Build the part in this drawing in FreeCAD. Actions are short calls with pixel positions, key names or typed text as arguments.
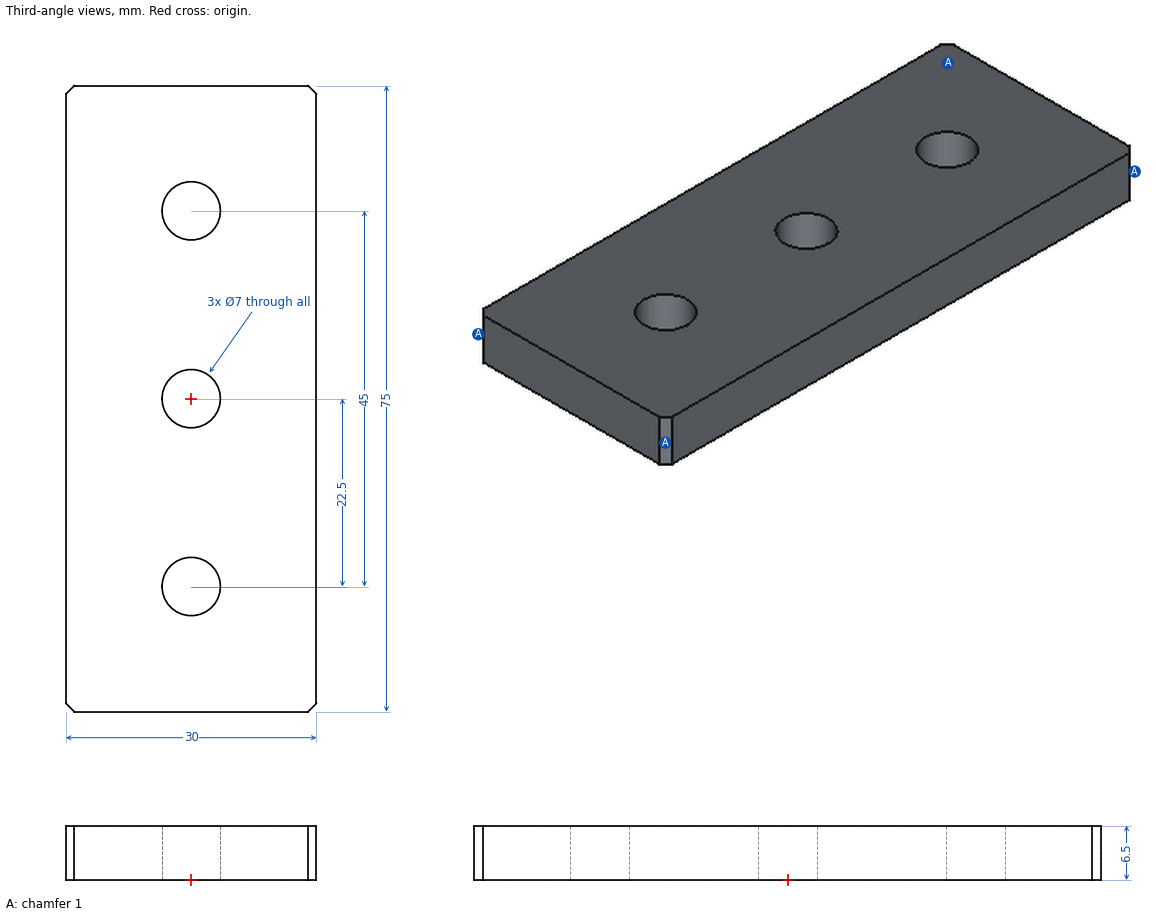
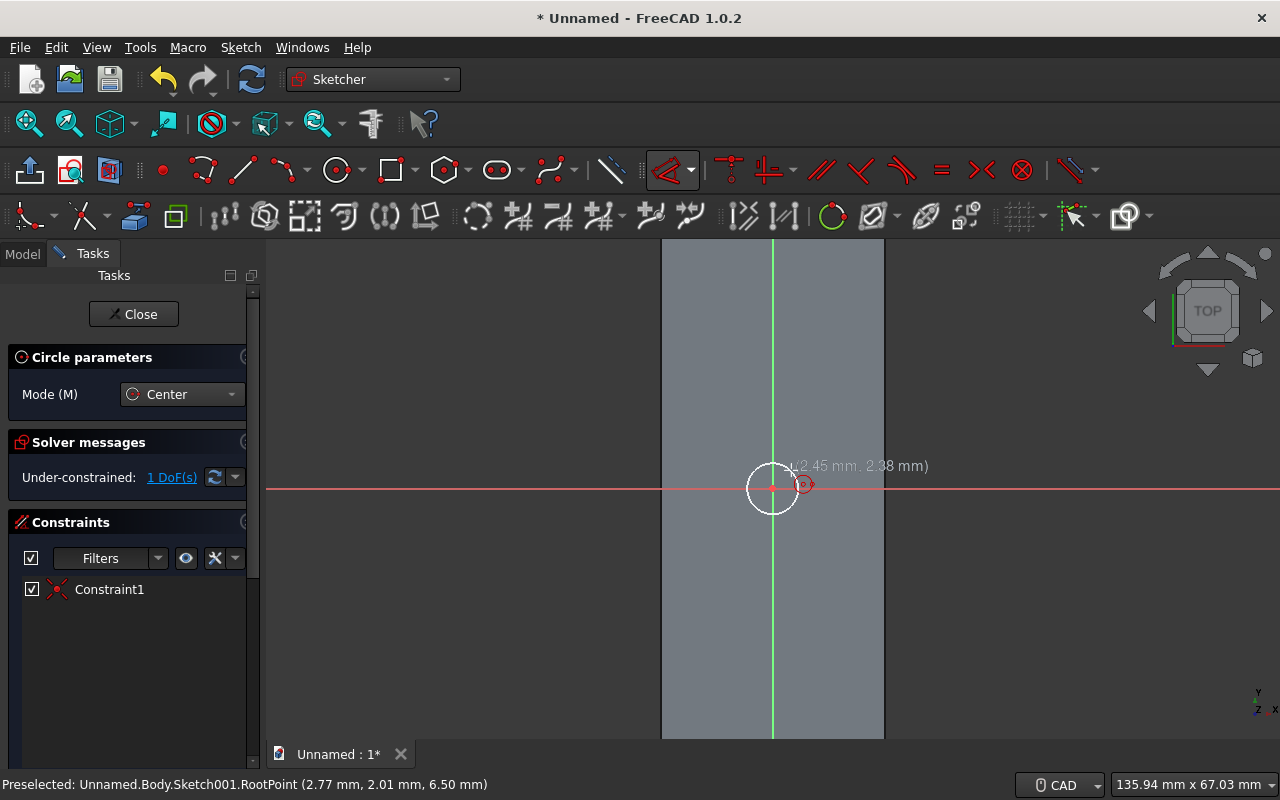
click(773, 657)
click(791, 638)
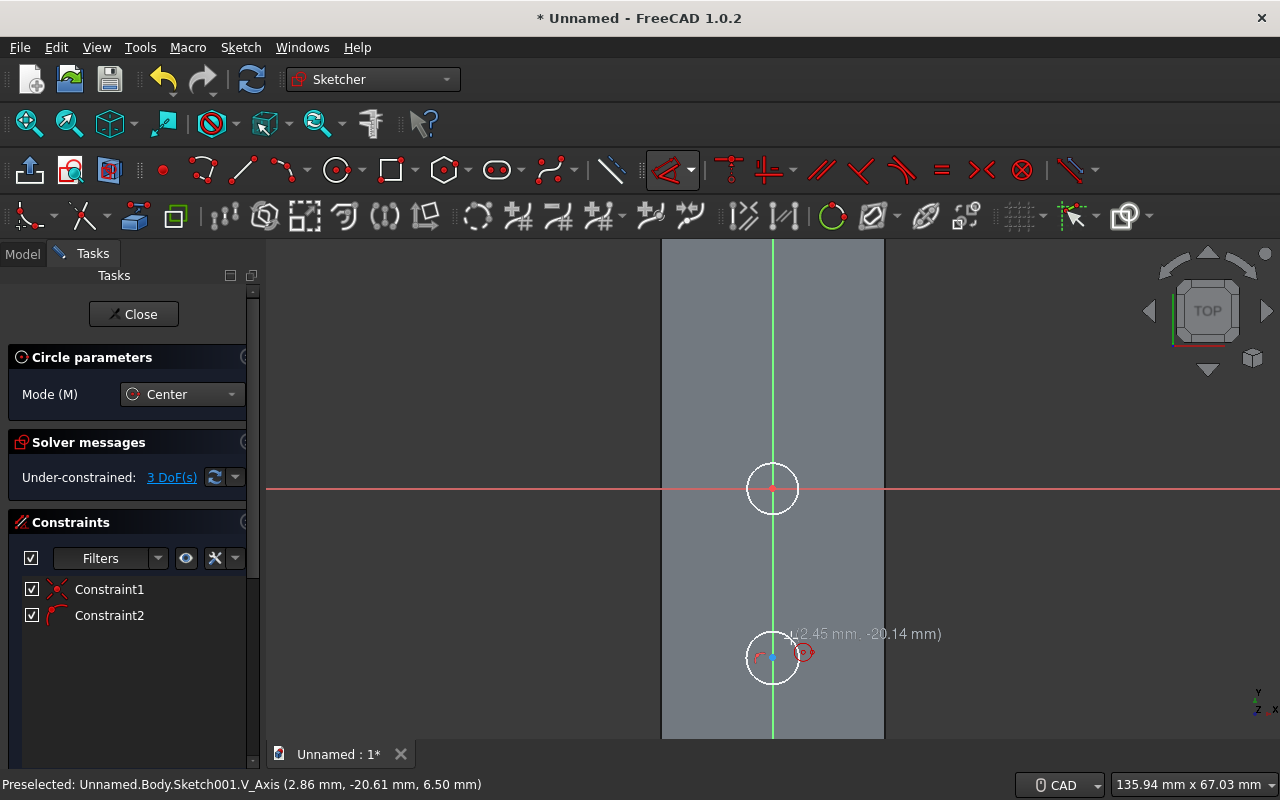
click(773, 321)
click(791, 302)
key(Escape)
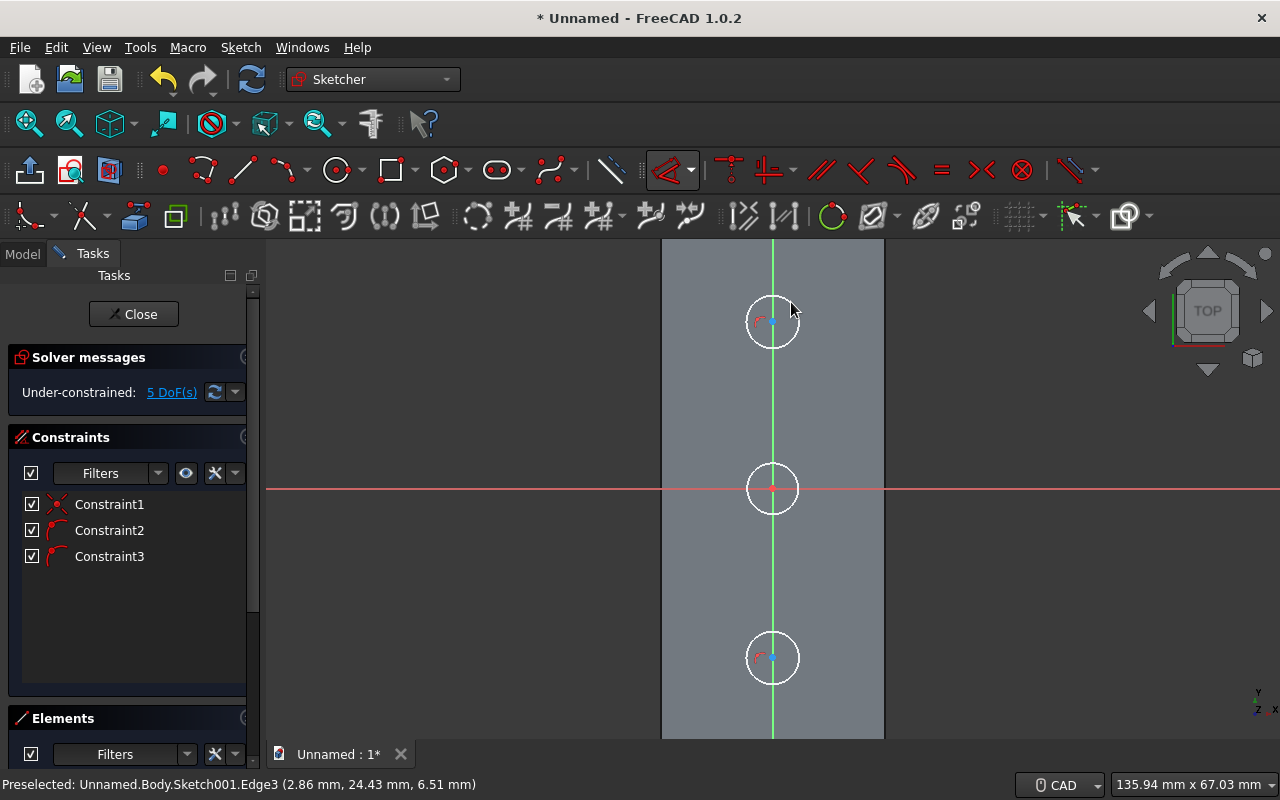
click(791, 471)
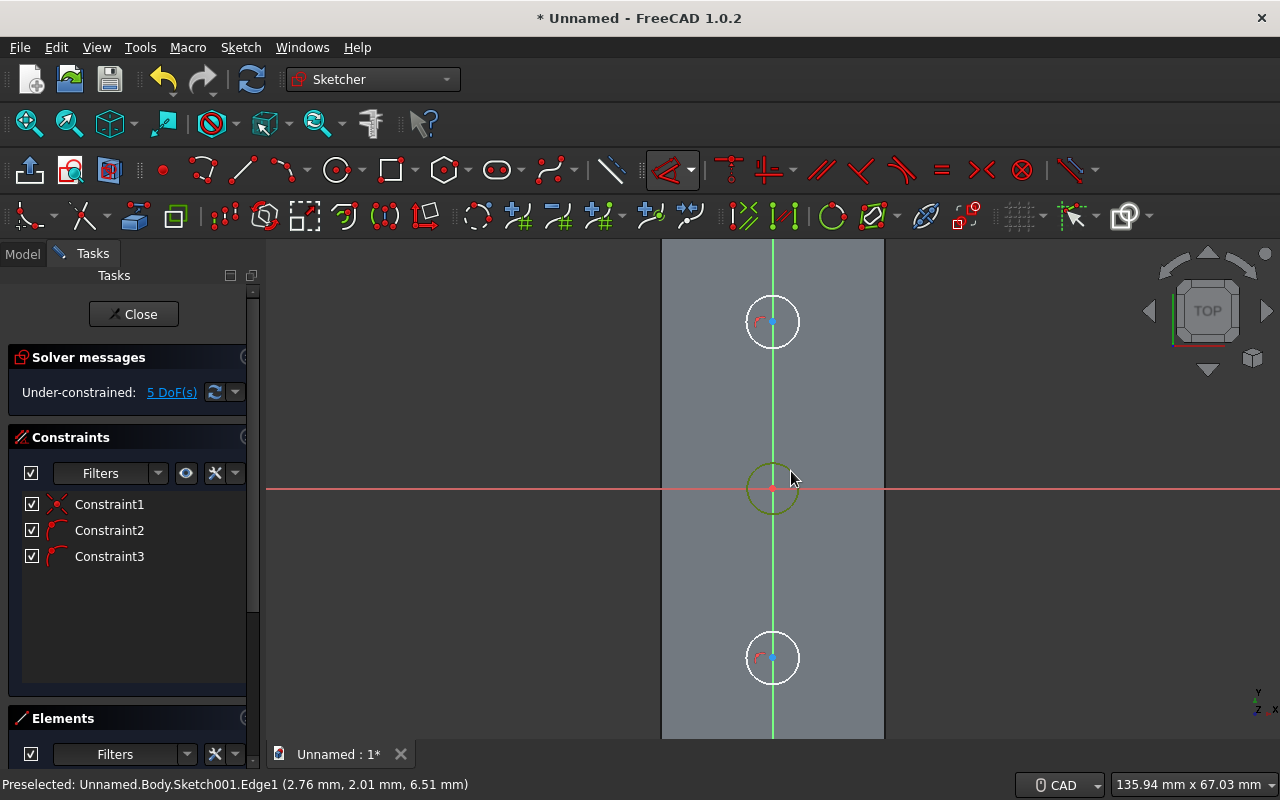
click(791, 639)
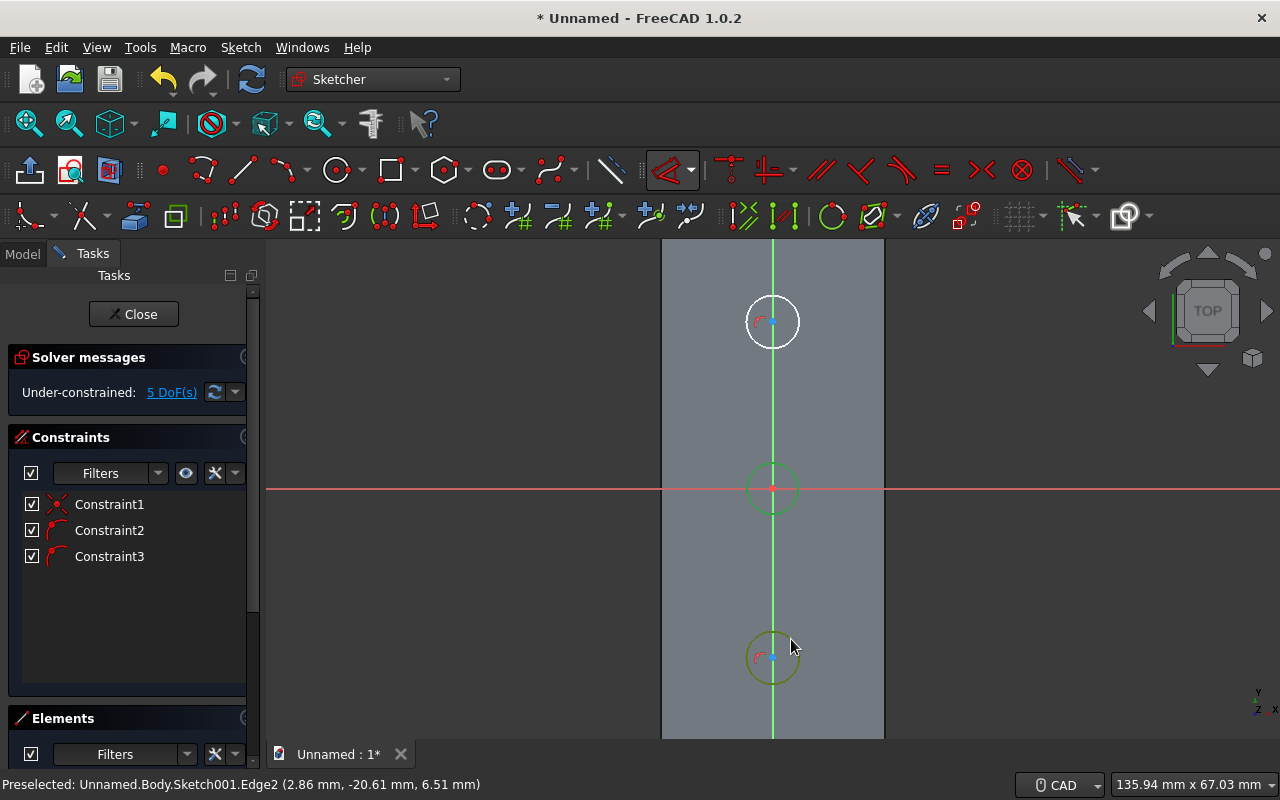
click(791, 303)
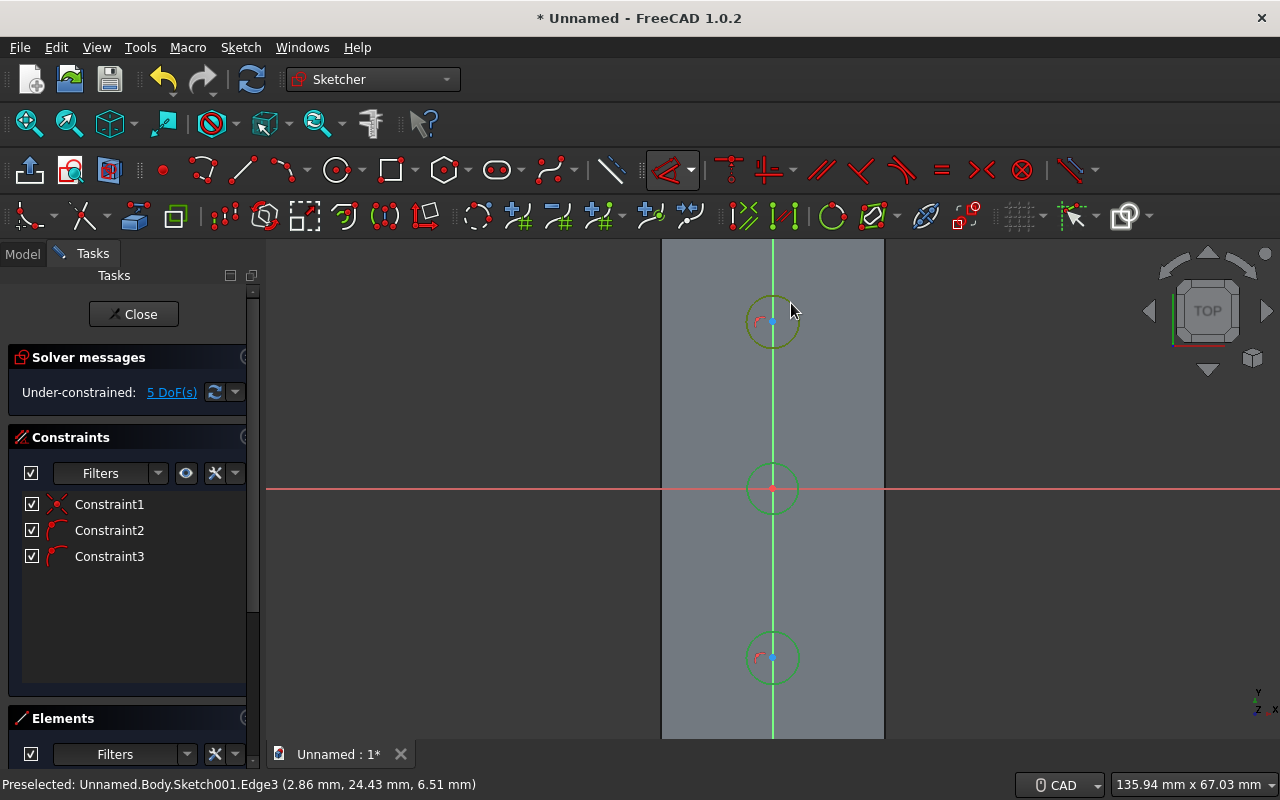
click(942, 170)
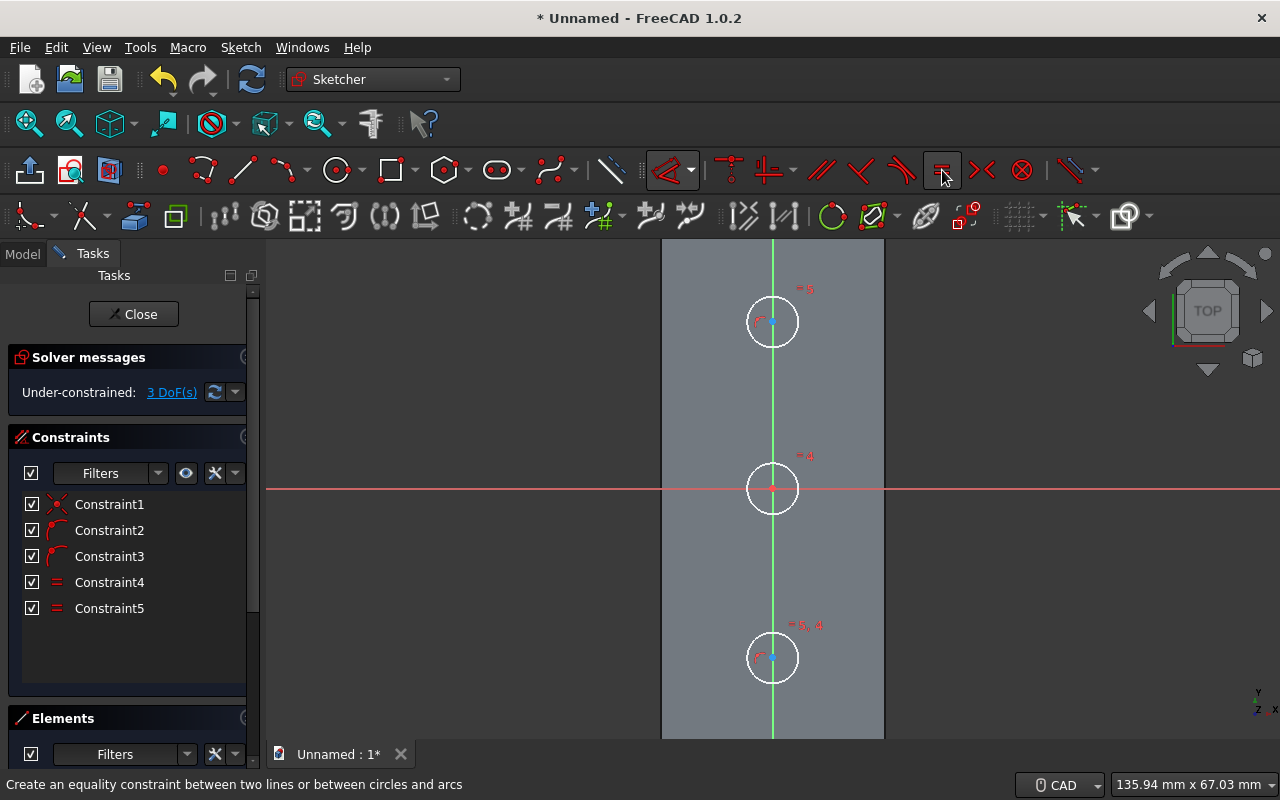
key(d)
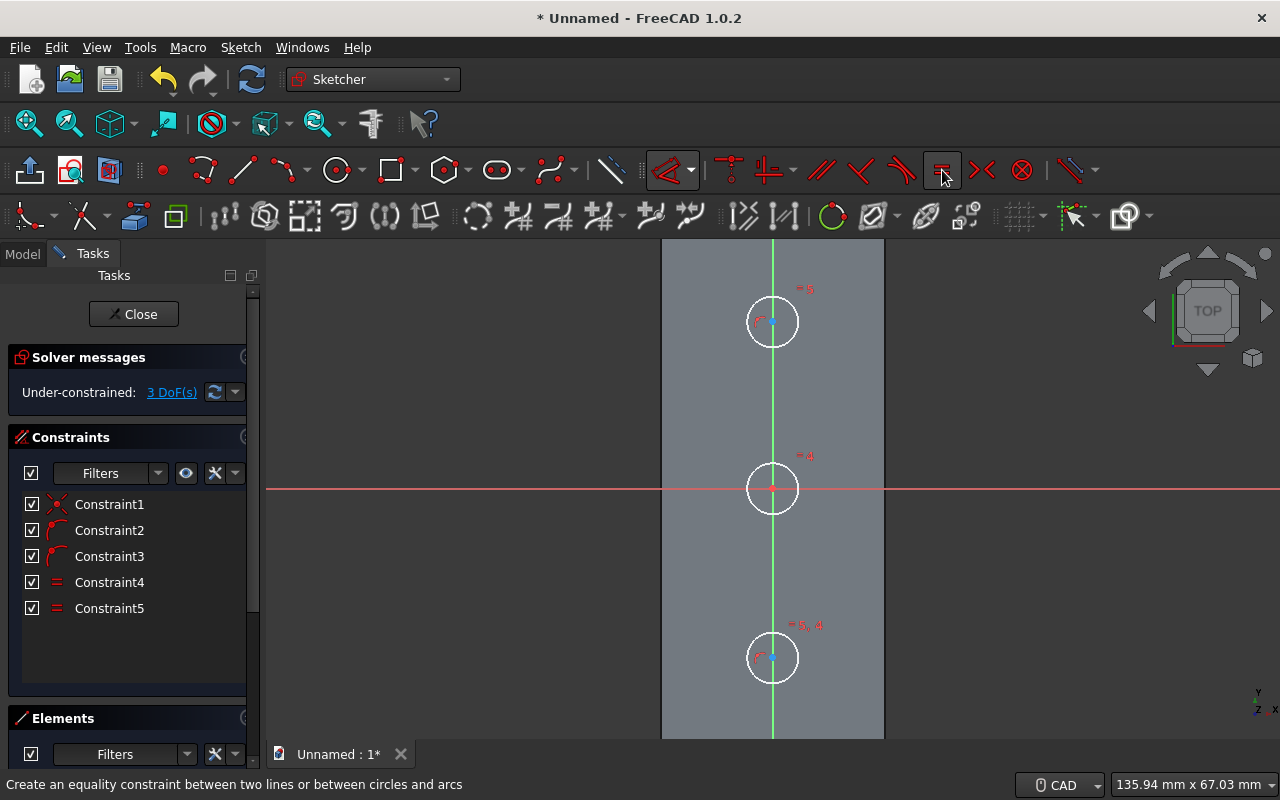
click(791, 471)
click(814, 449)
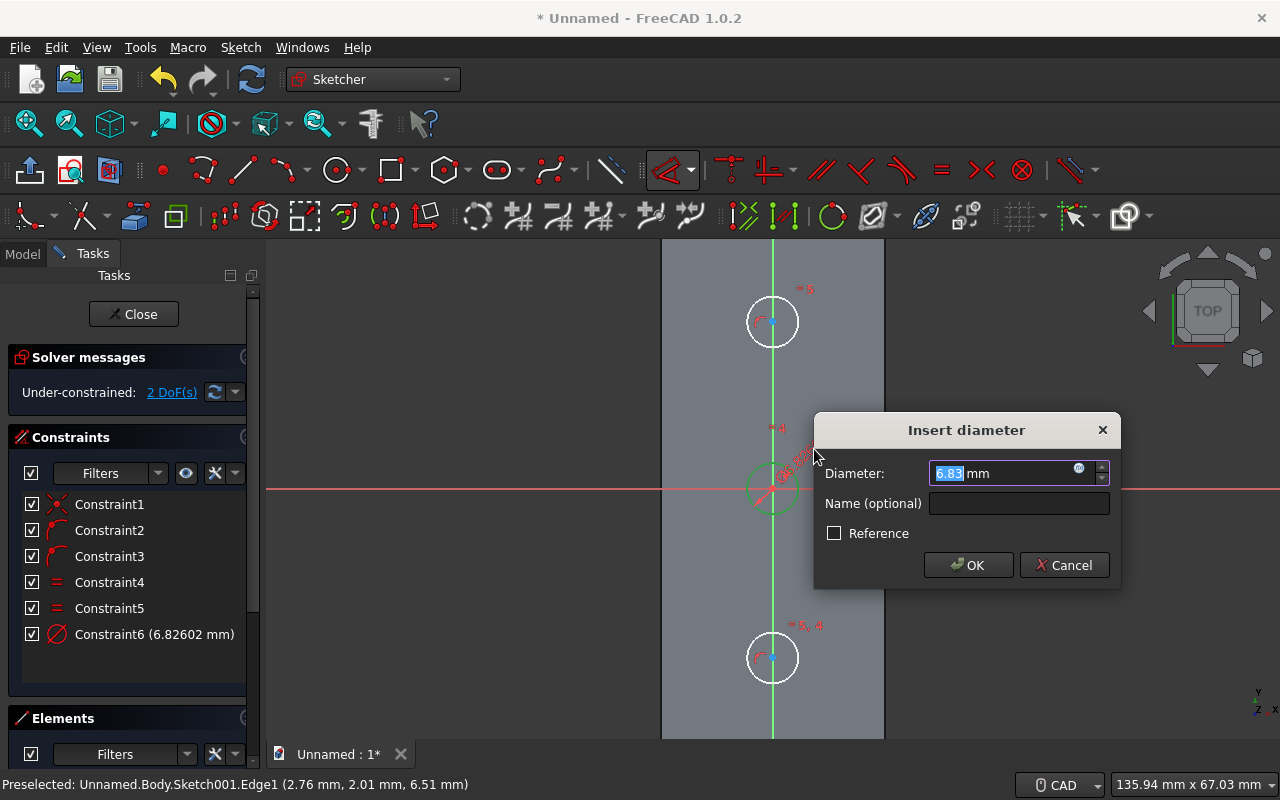
text(7)
key(Return)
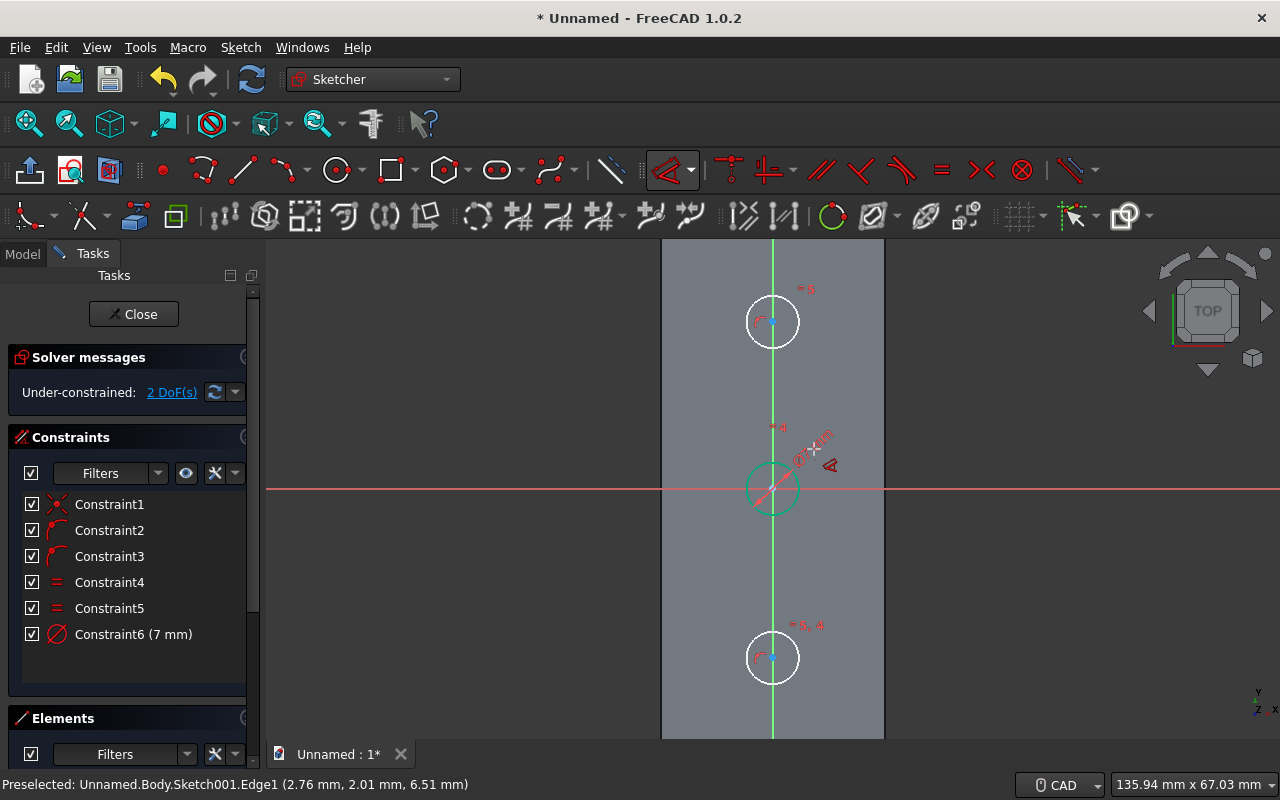
click(773, 658)